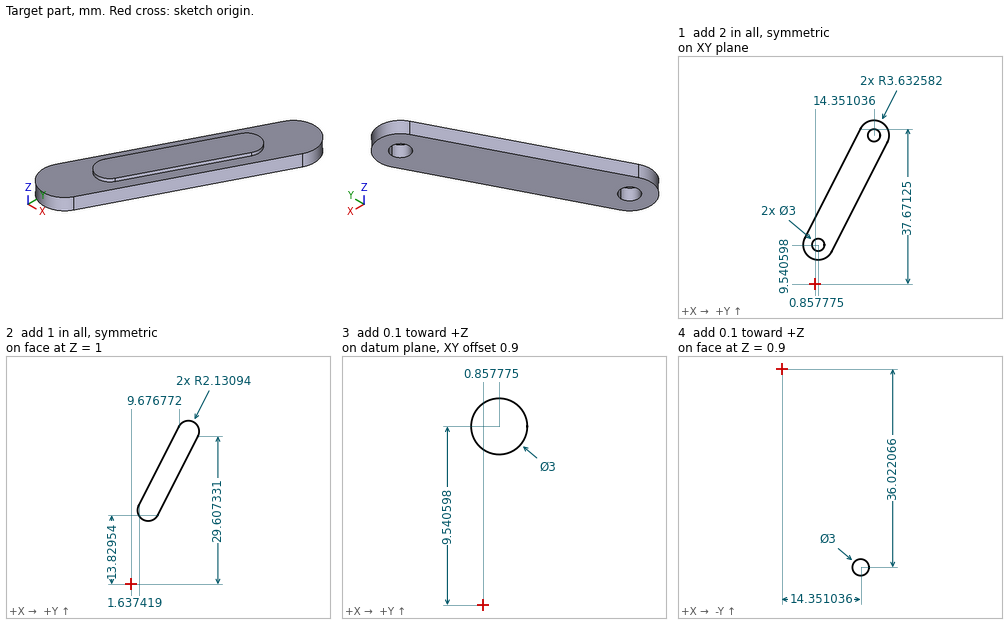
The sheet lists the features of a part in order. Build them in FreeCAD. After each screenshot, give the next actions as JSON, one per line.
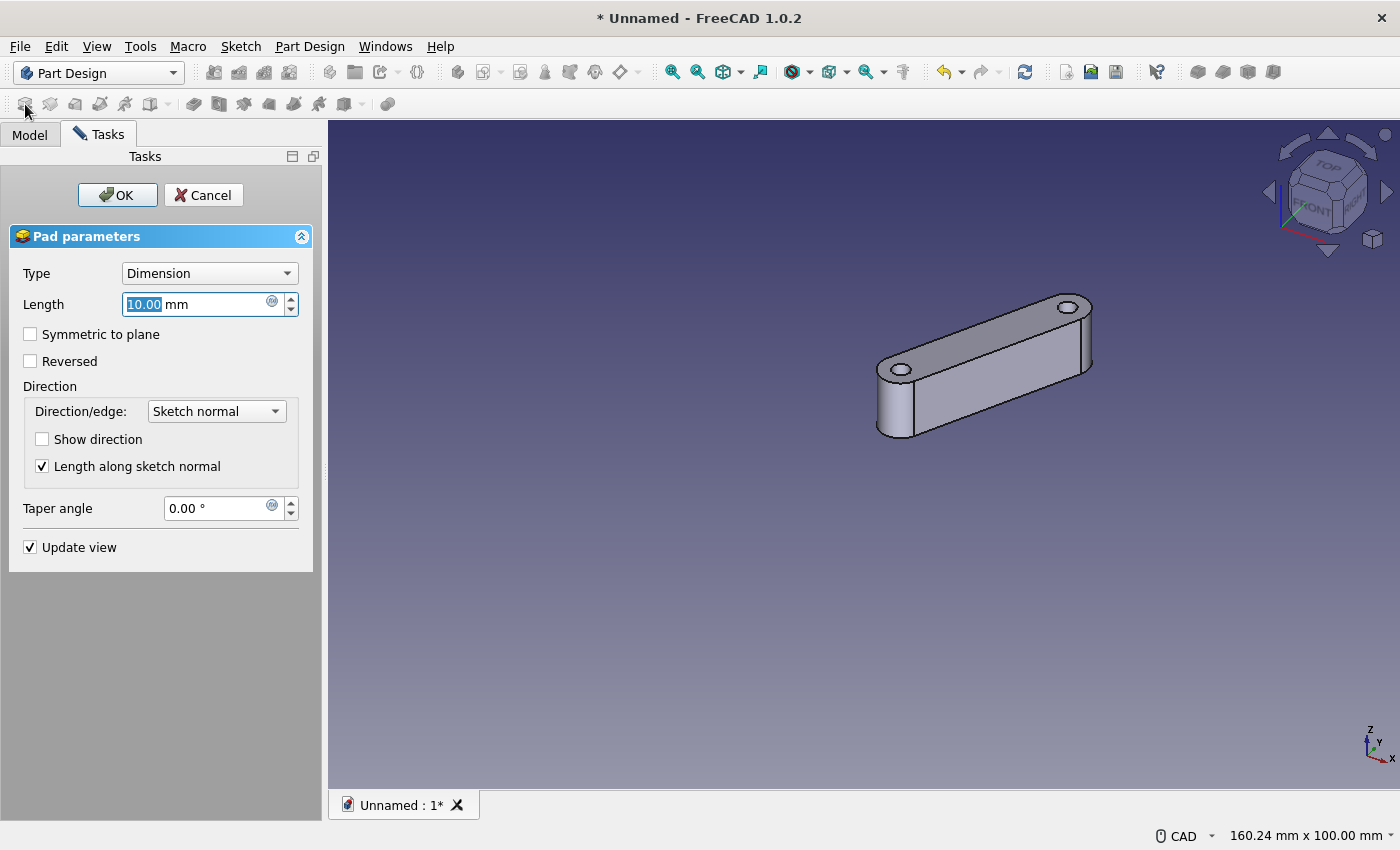
{"action": "type", "text": "2"}
{"action": "key", "text": "Tab"}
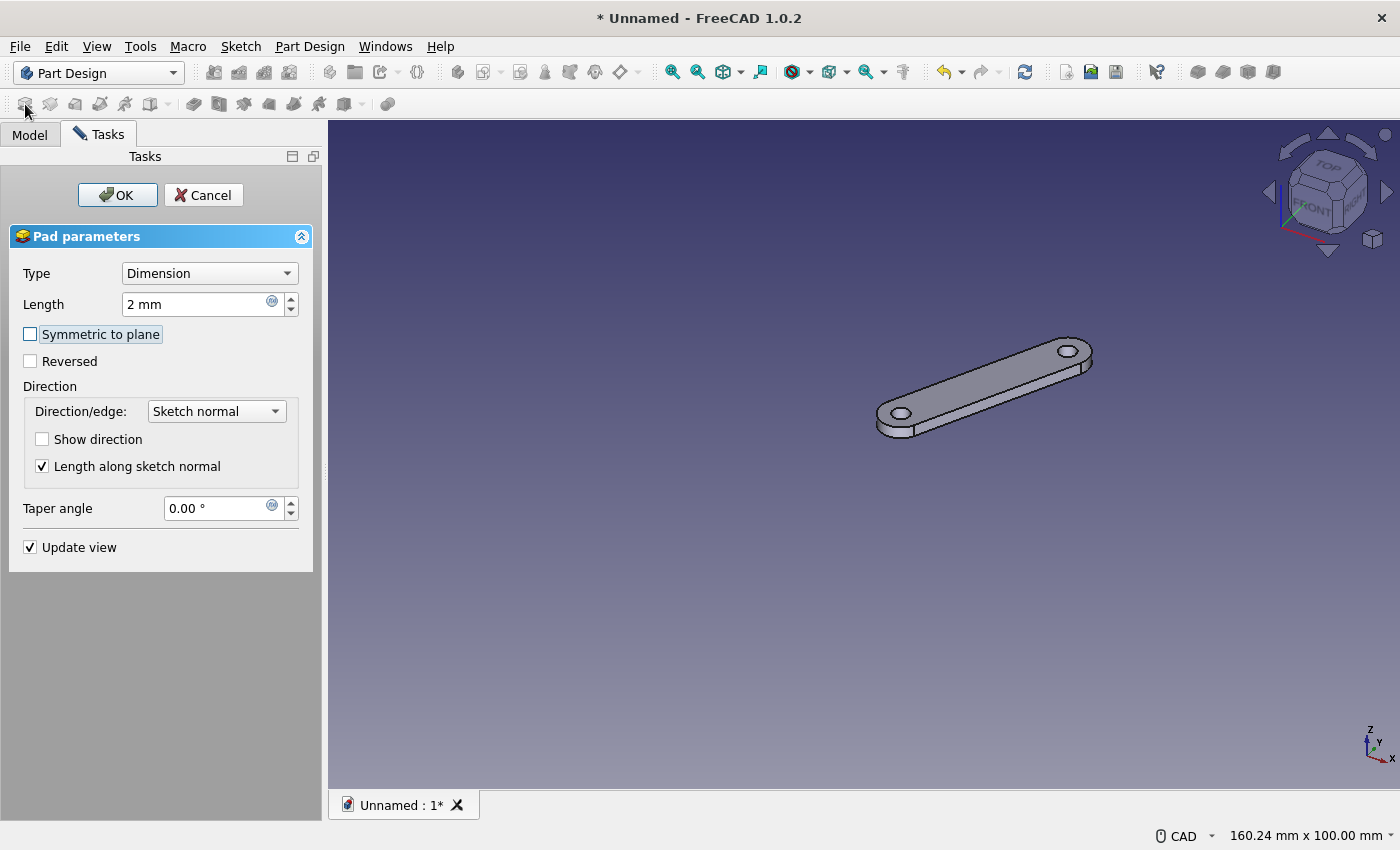
{"action": "left_click", "coordinate": [31, 334]}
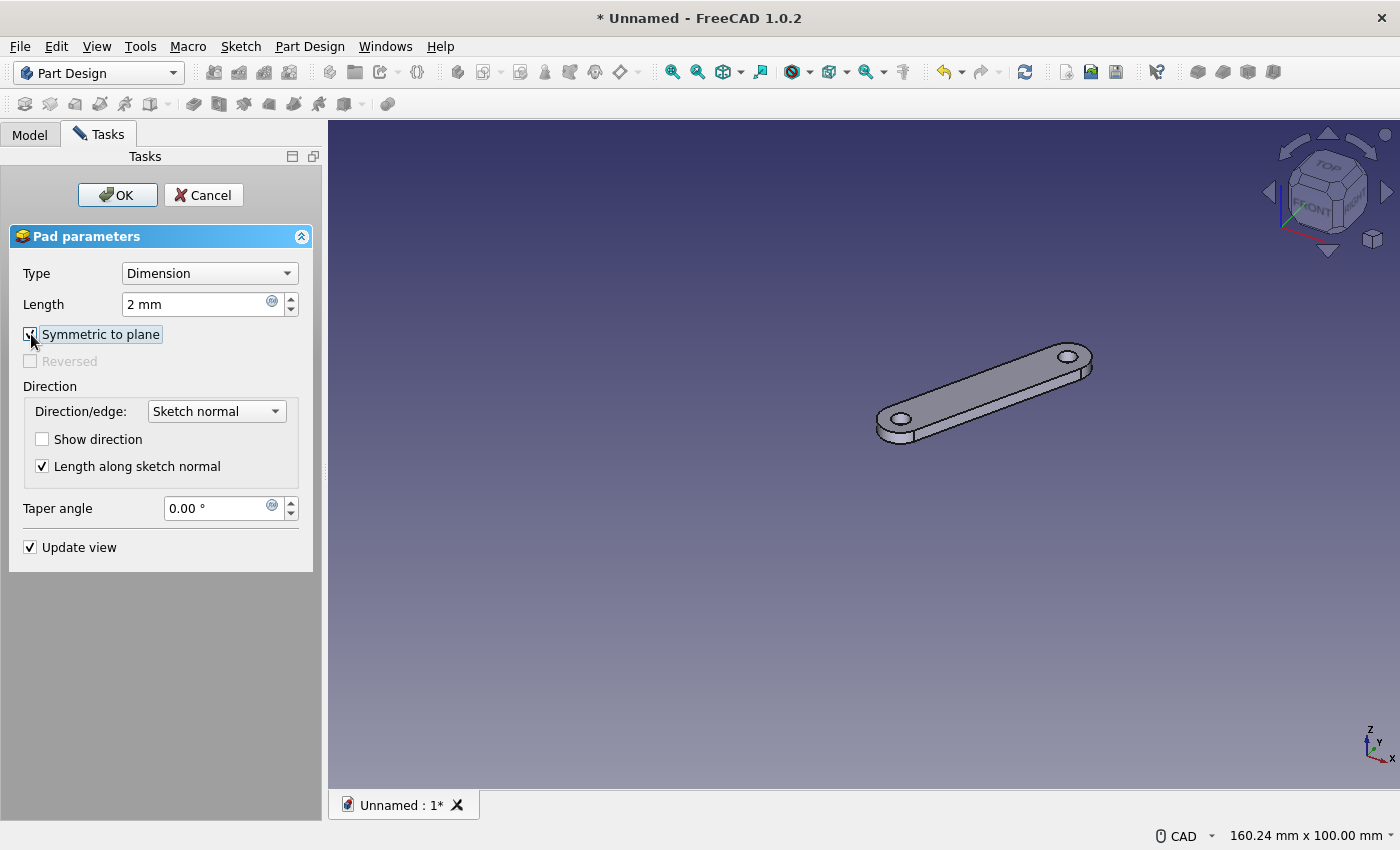
{"action": "left_click", "coordinate": [118, 195]}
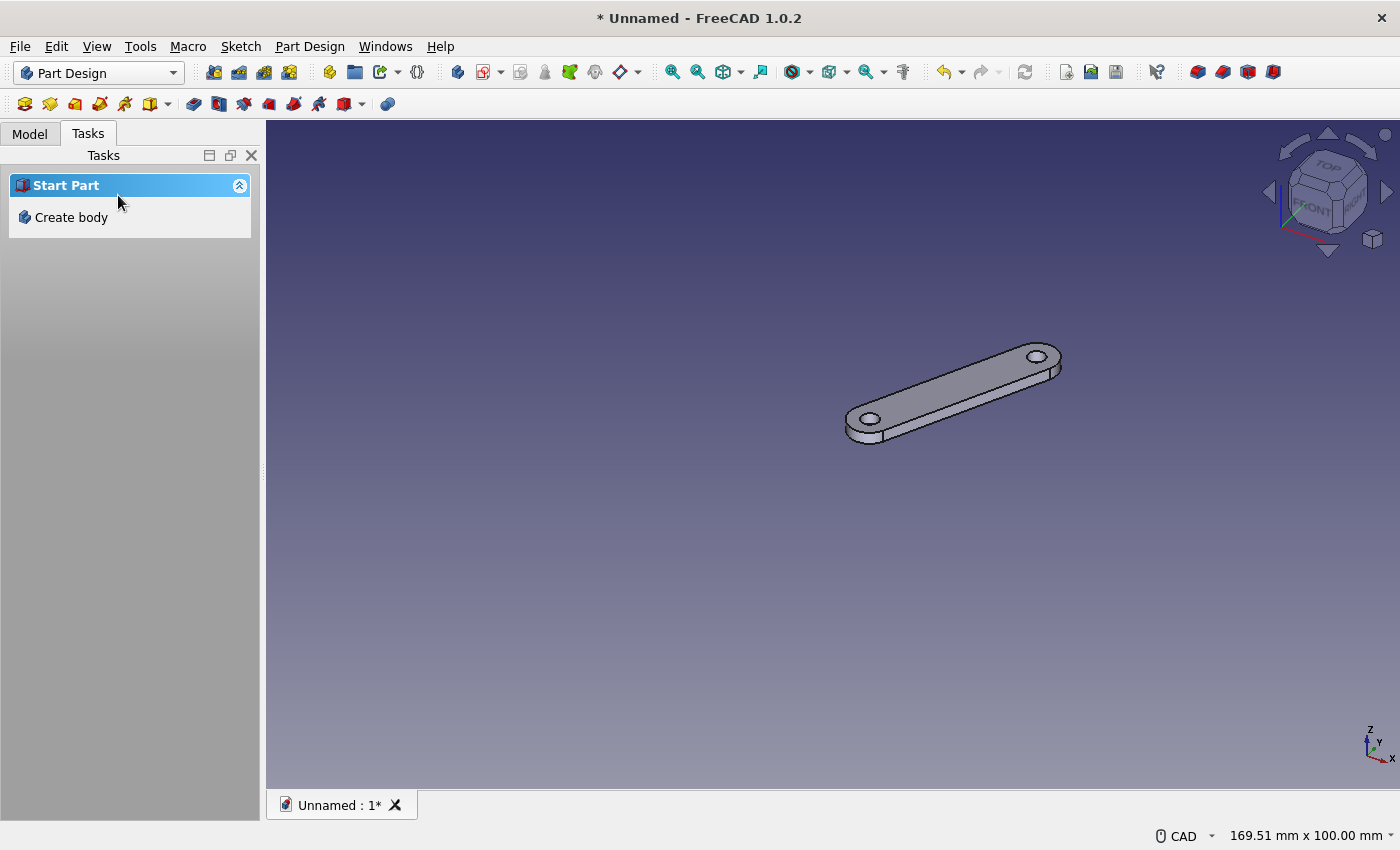
{"action": "key", "text": "v f"}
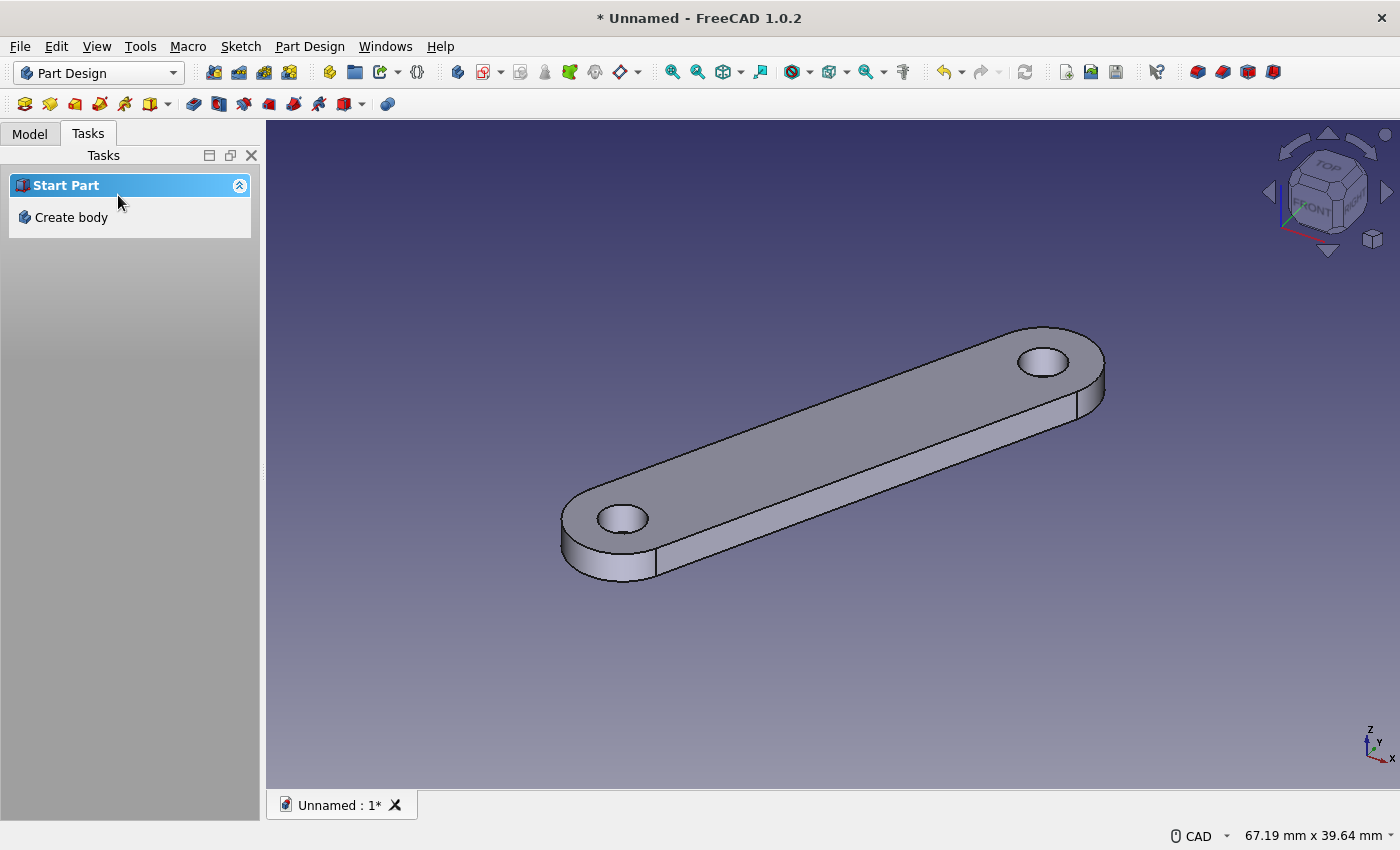
{"action": "left_click", "coordinate": [833, 440]}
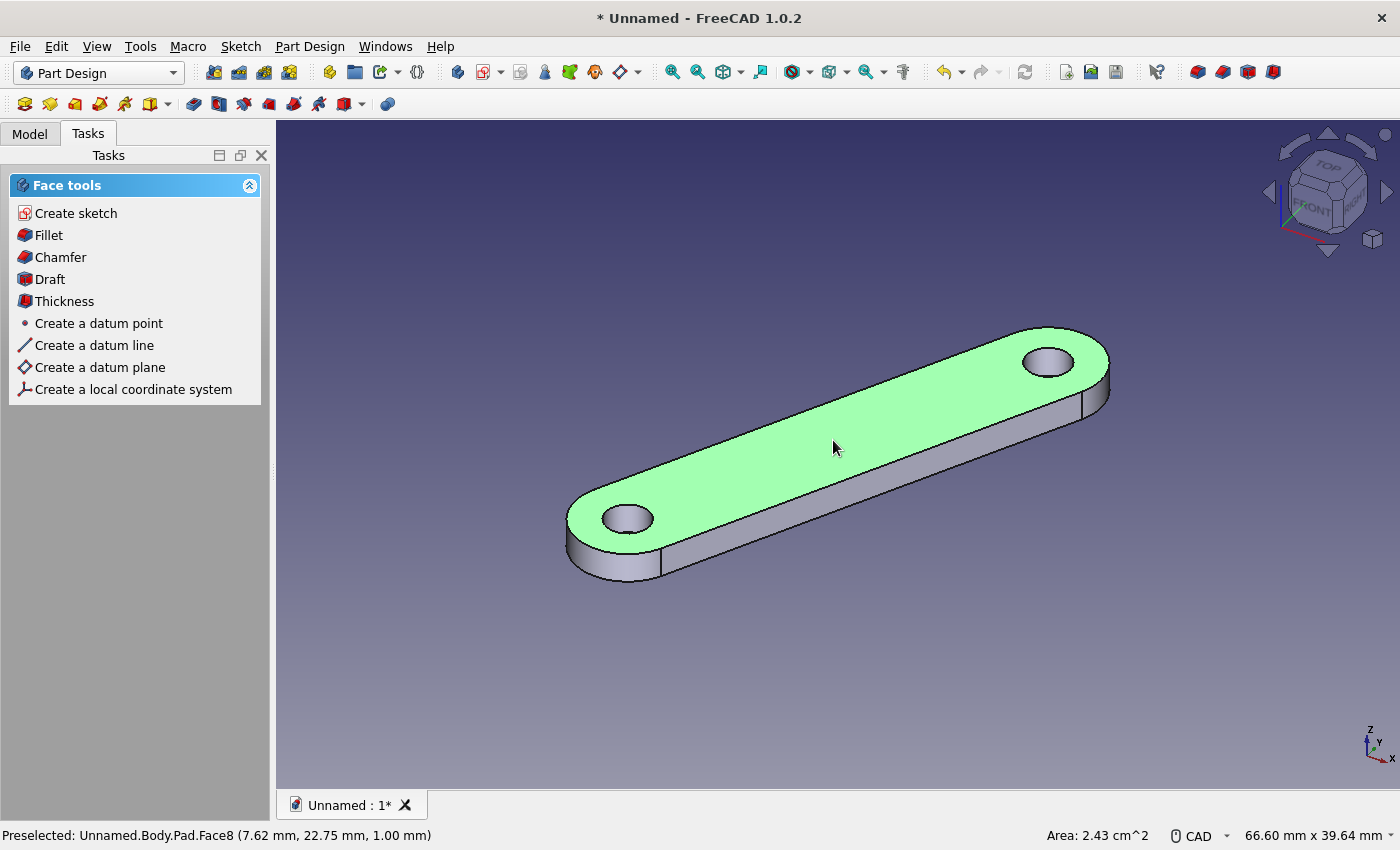
{"action": "left_click", "coordinate": [482, 72]}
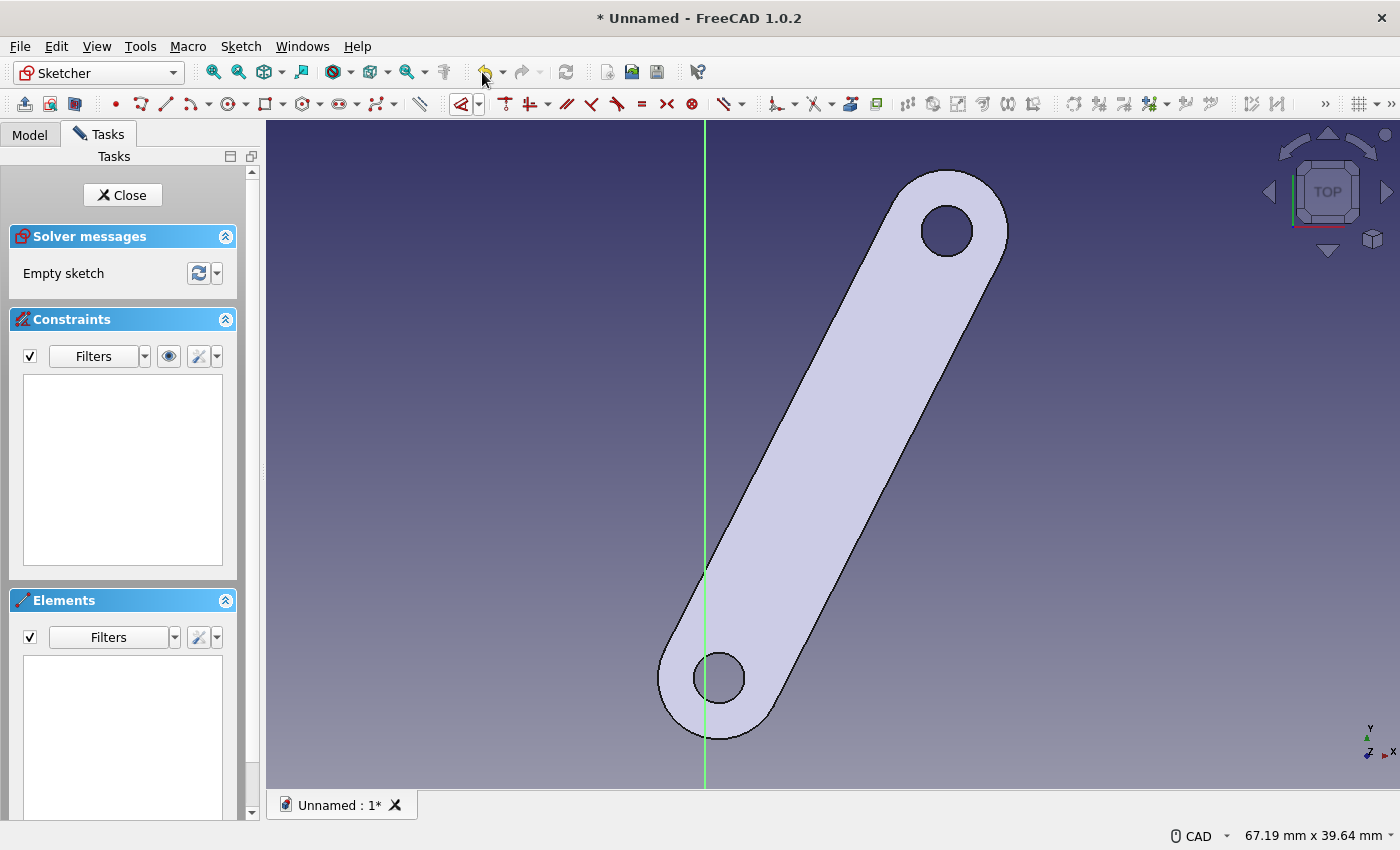
{"action": "scroll", "coordinate": [521, 148], "scroll_direction": "down", "scroll_amount": 1}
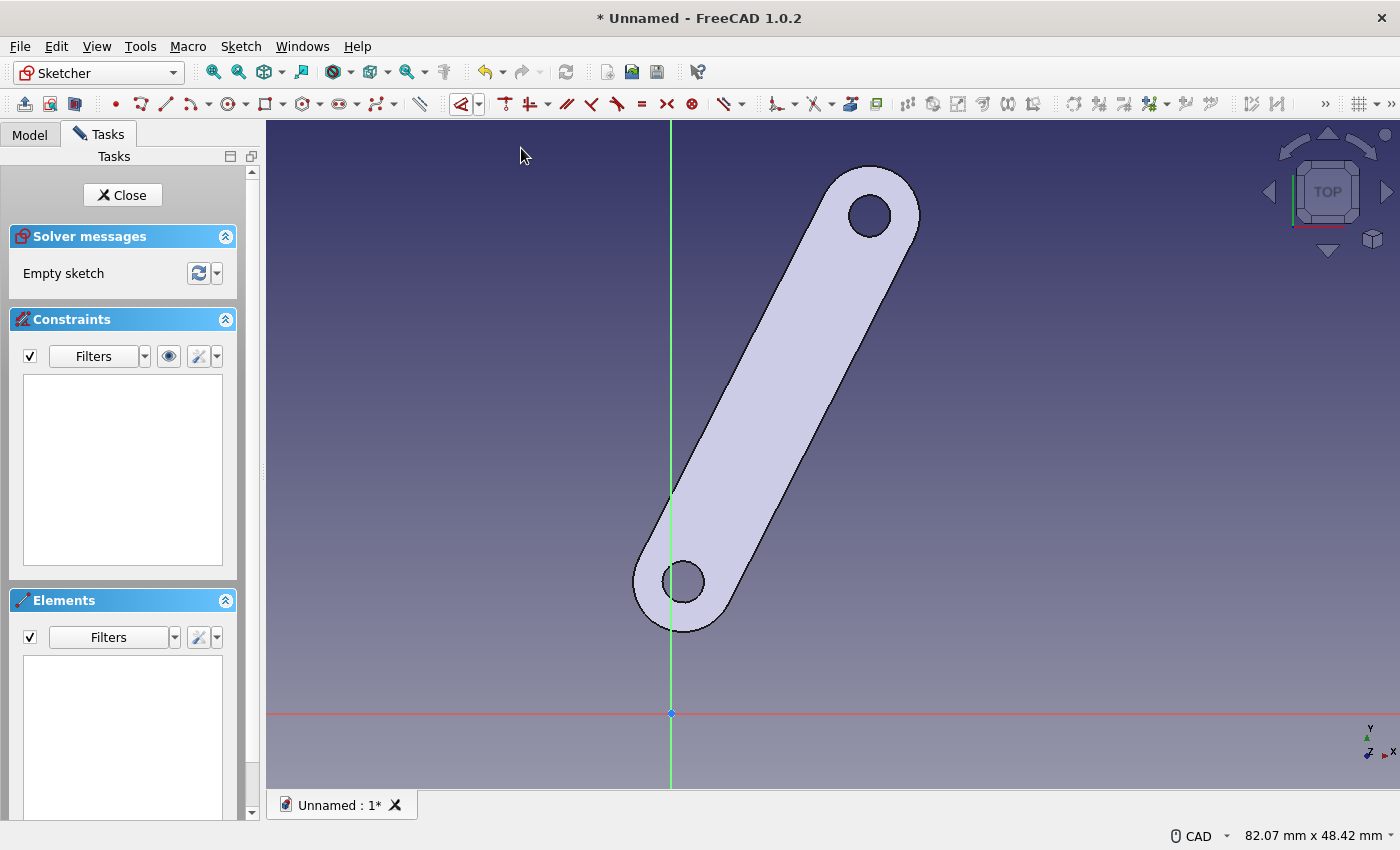
{"action": "key", "text": "g s"}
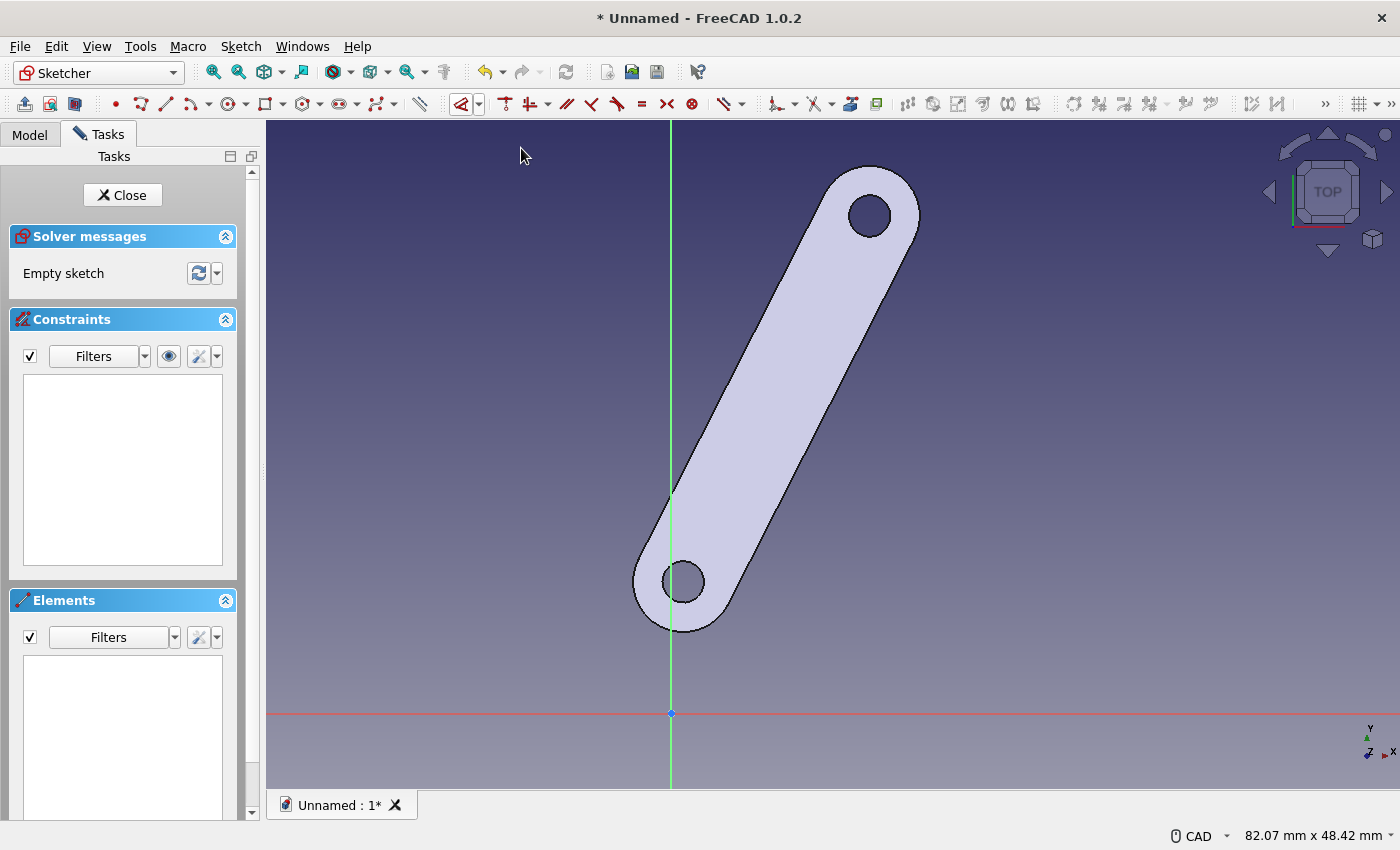
{"action": "left_click", "coordinate": [720, 509]}